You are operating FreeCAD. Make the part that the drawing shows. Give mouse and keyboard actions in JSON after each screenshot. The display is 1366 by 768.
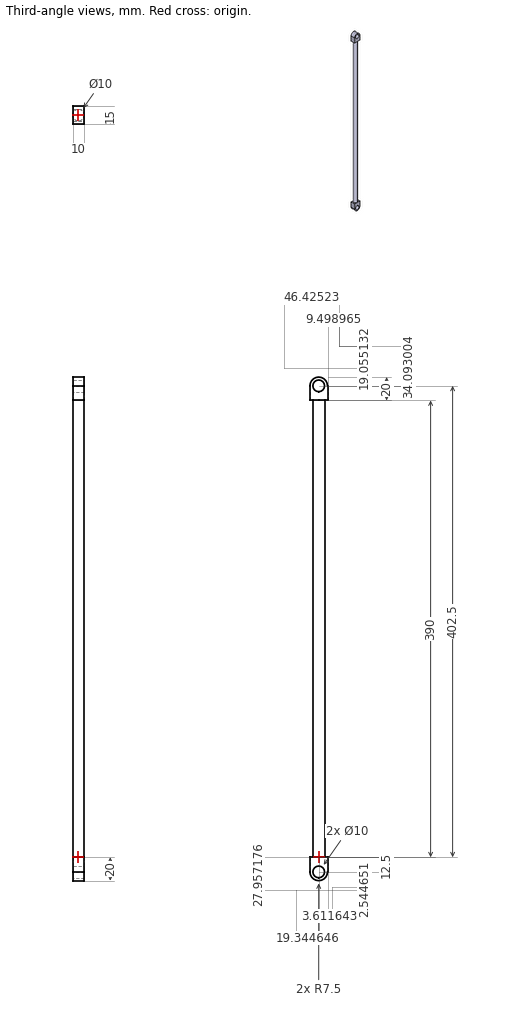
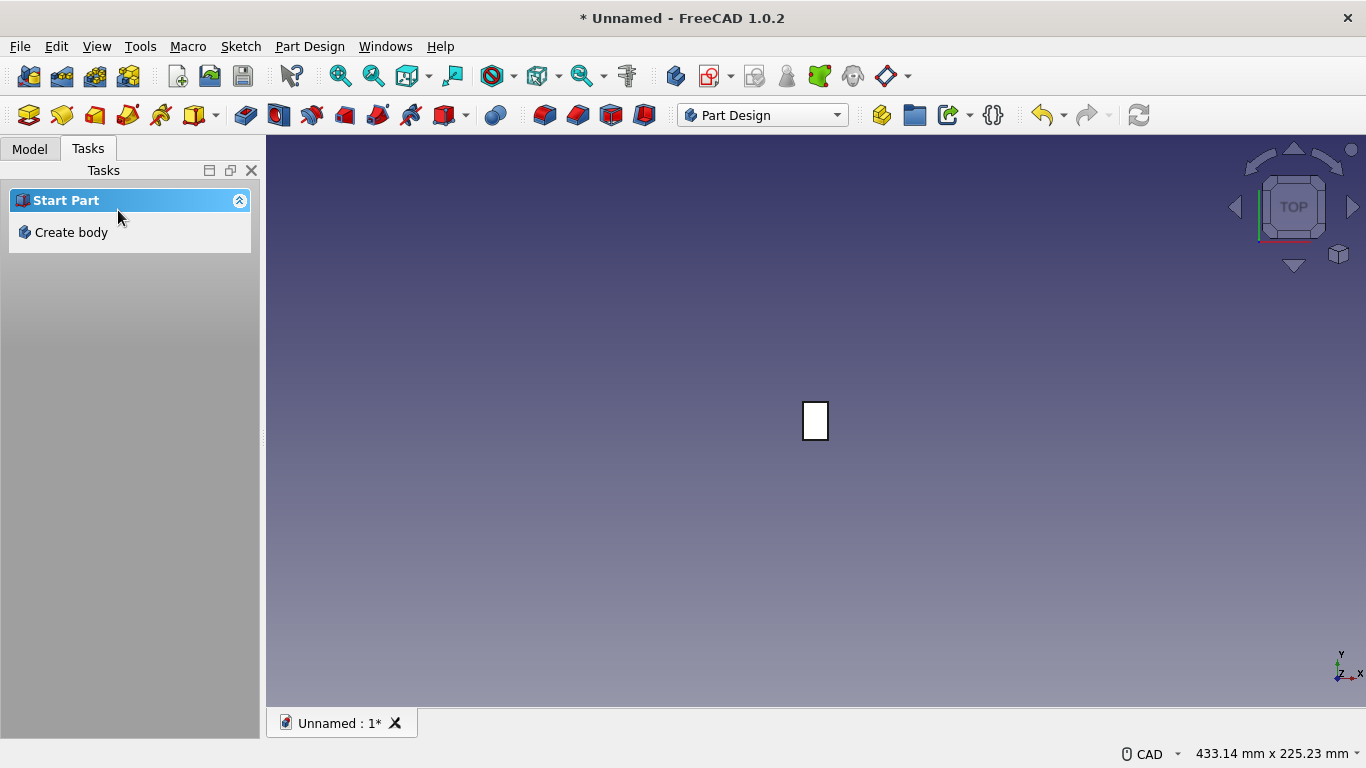
{"action": "left_click", "coordinate": [341, 76]}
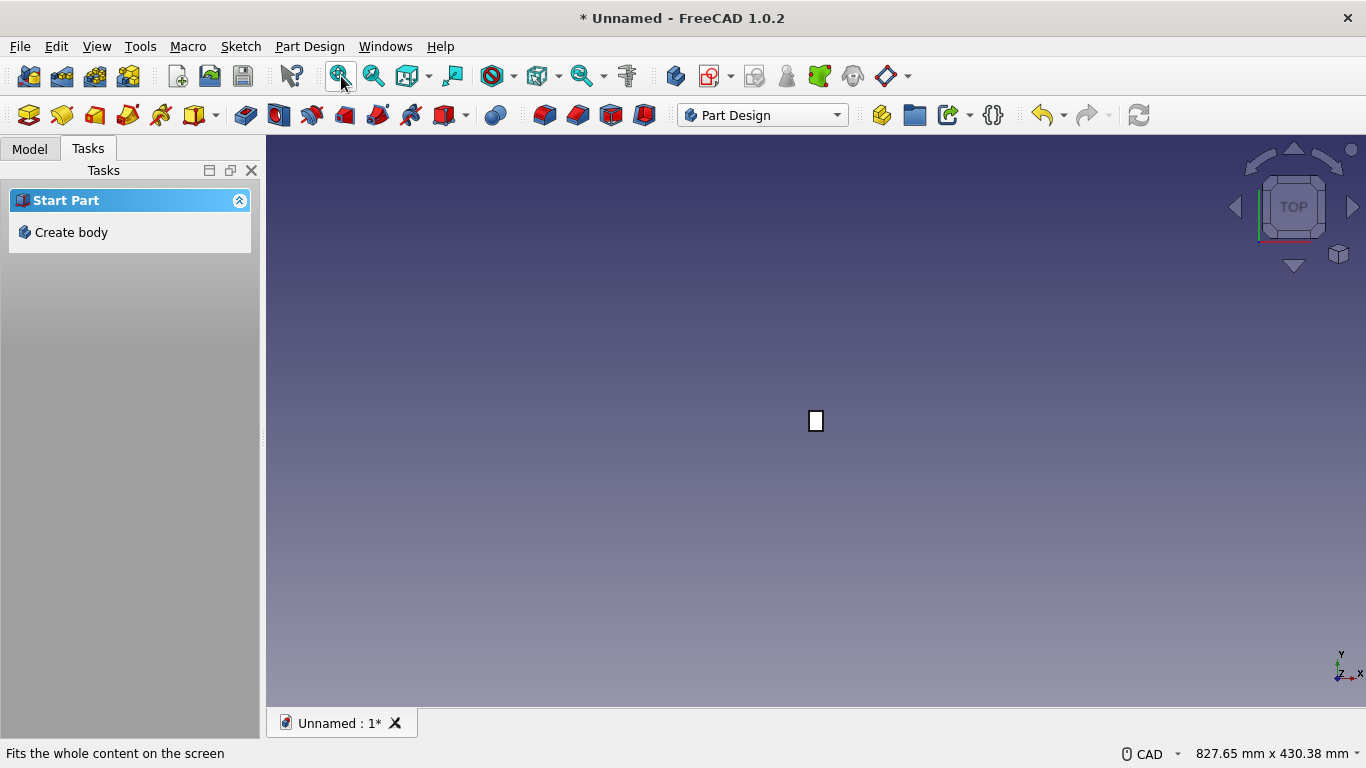
{"action": "key", "text": "0"}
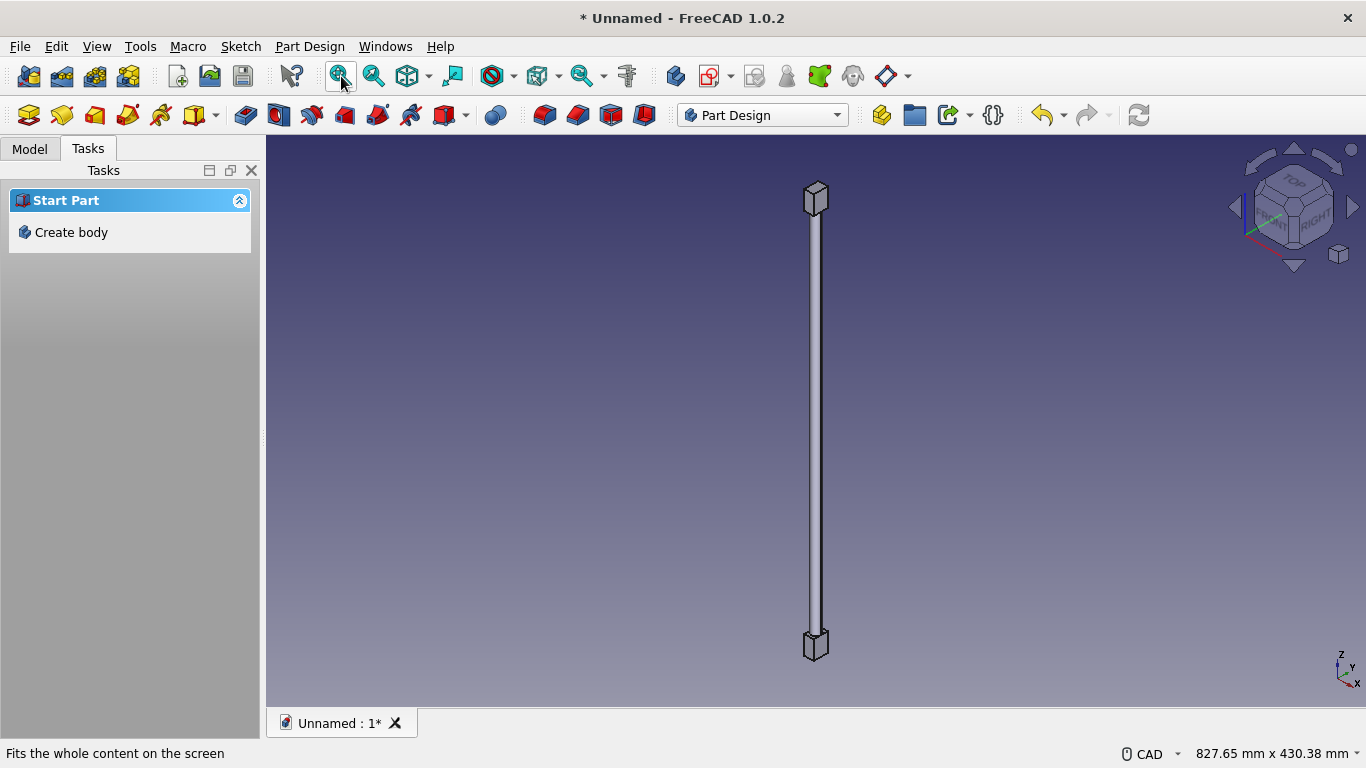
{"action": "left_click", "coordinate": [823, 199]}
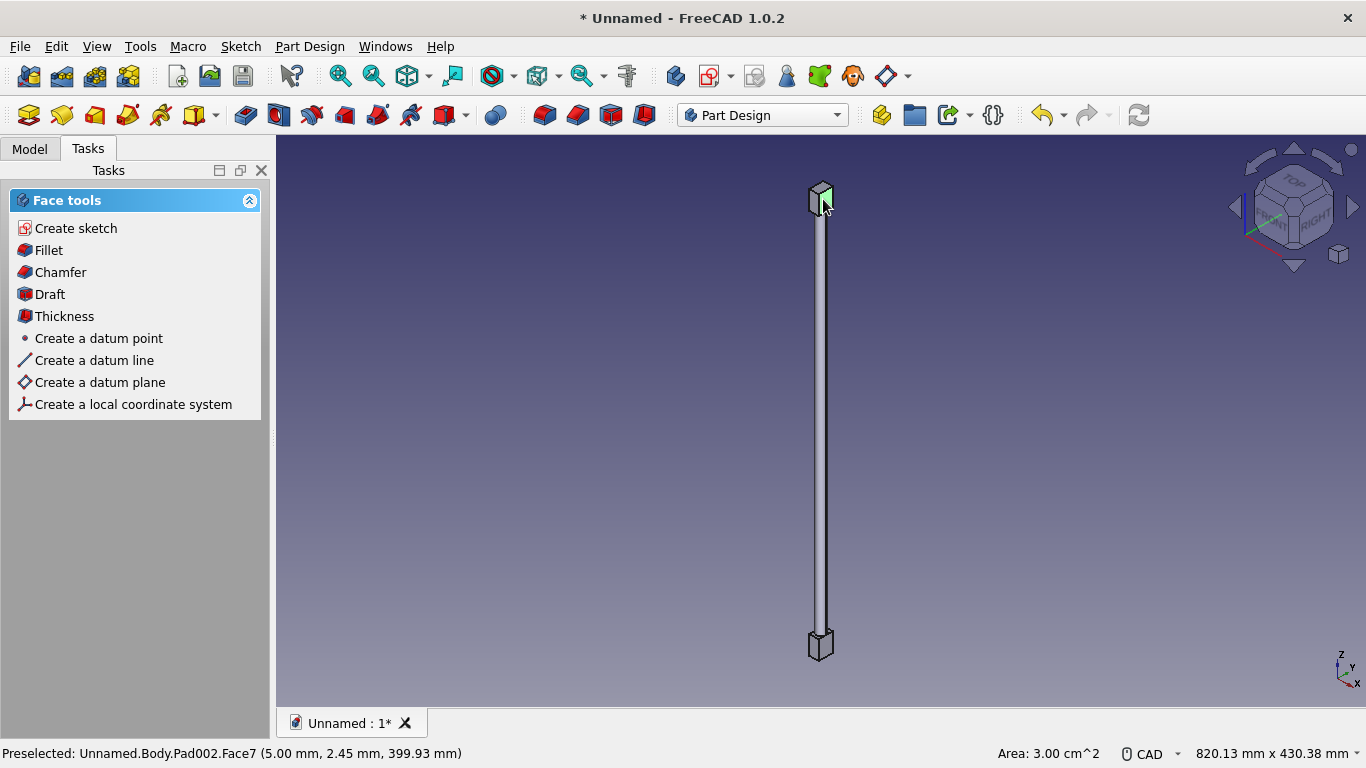
{"action": "left_click", "coordinate": [708, 76]}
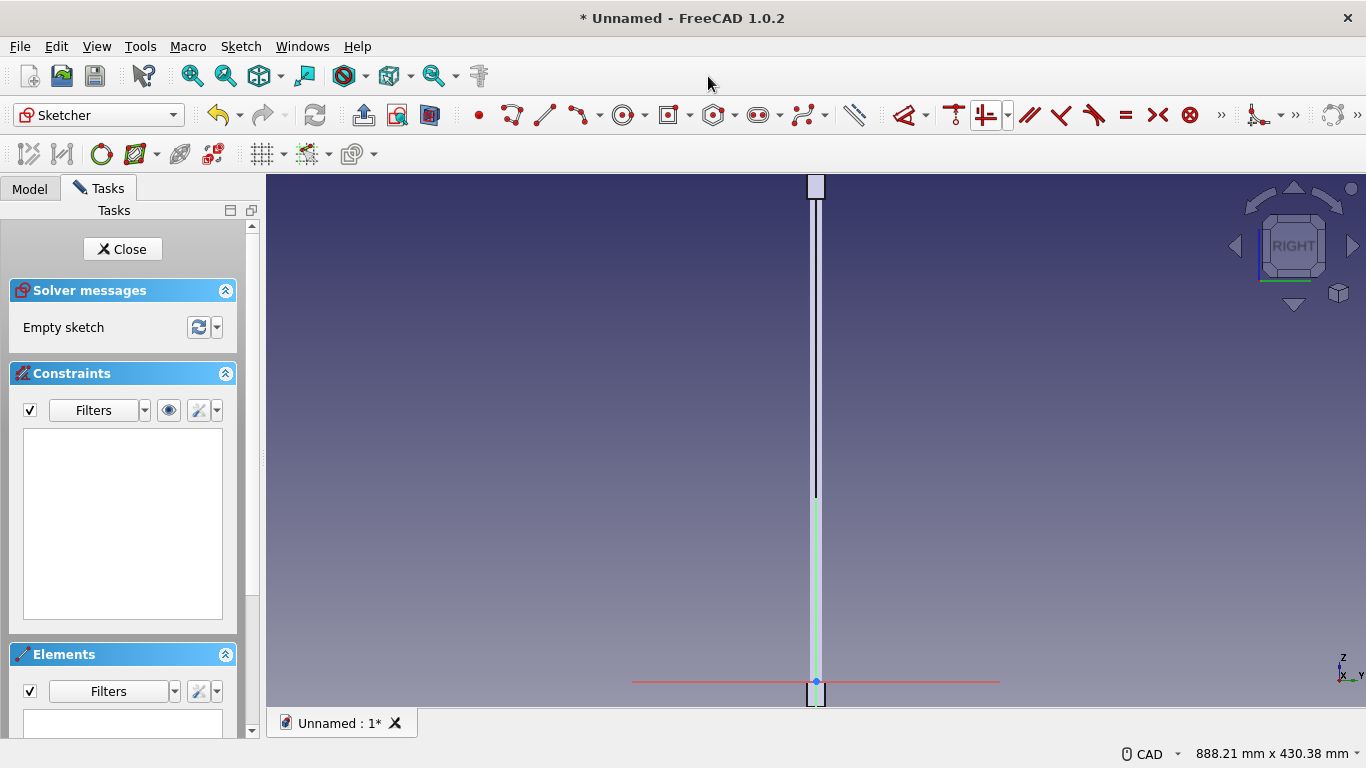
{"action": "scroll", "coordinate": [674, 455], "scroll_direction": "down", "scroll_amount": 3}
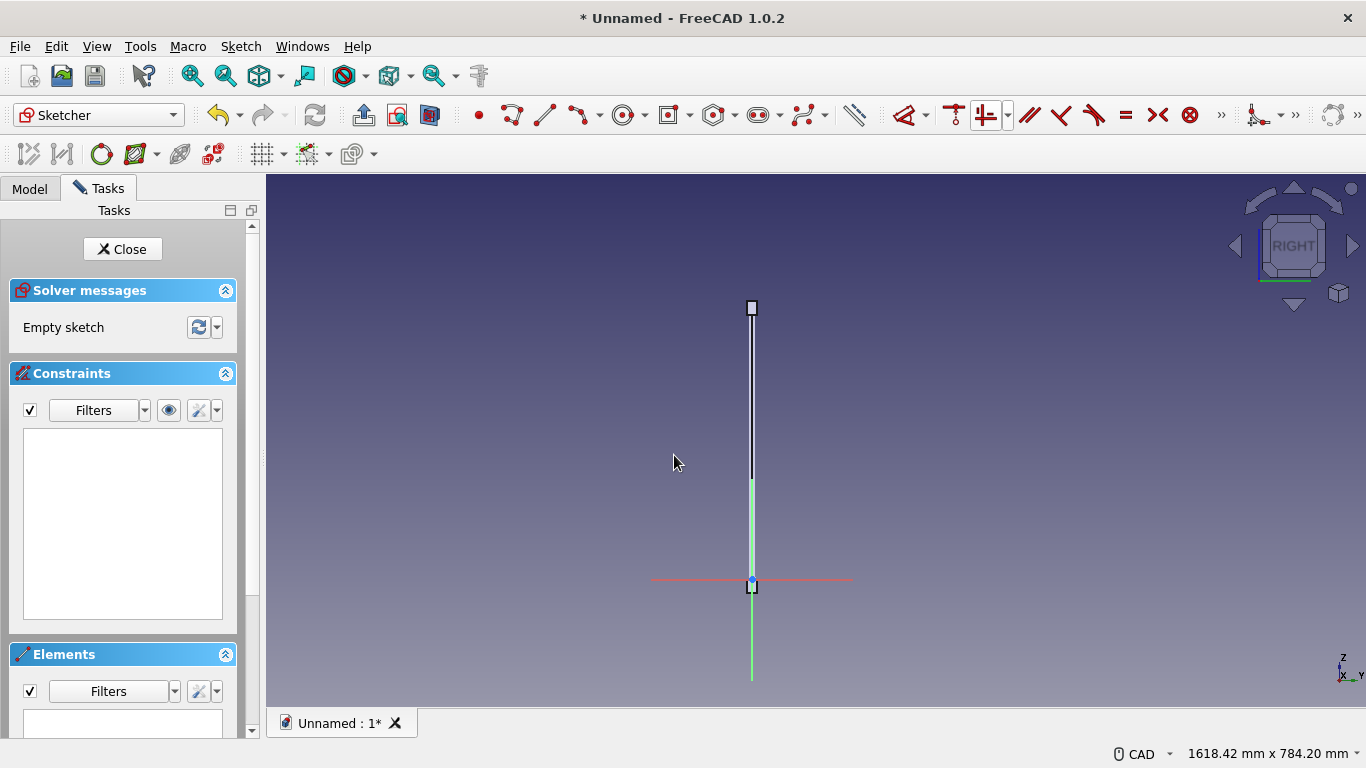
{"action": "left_click", "coordinate": [512, 116]}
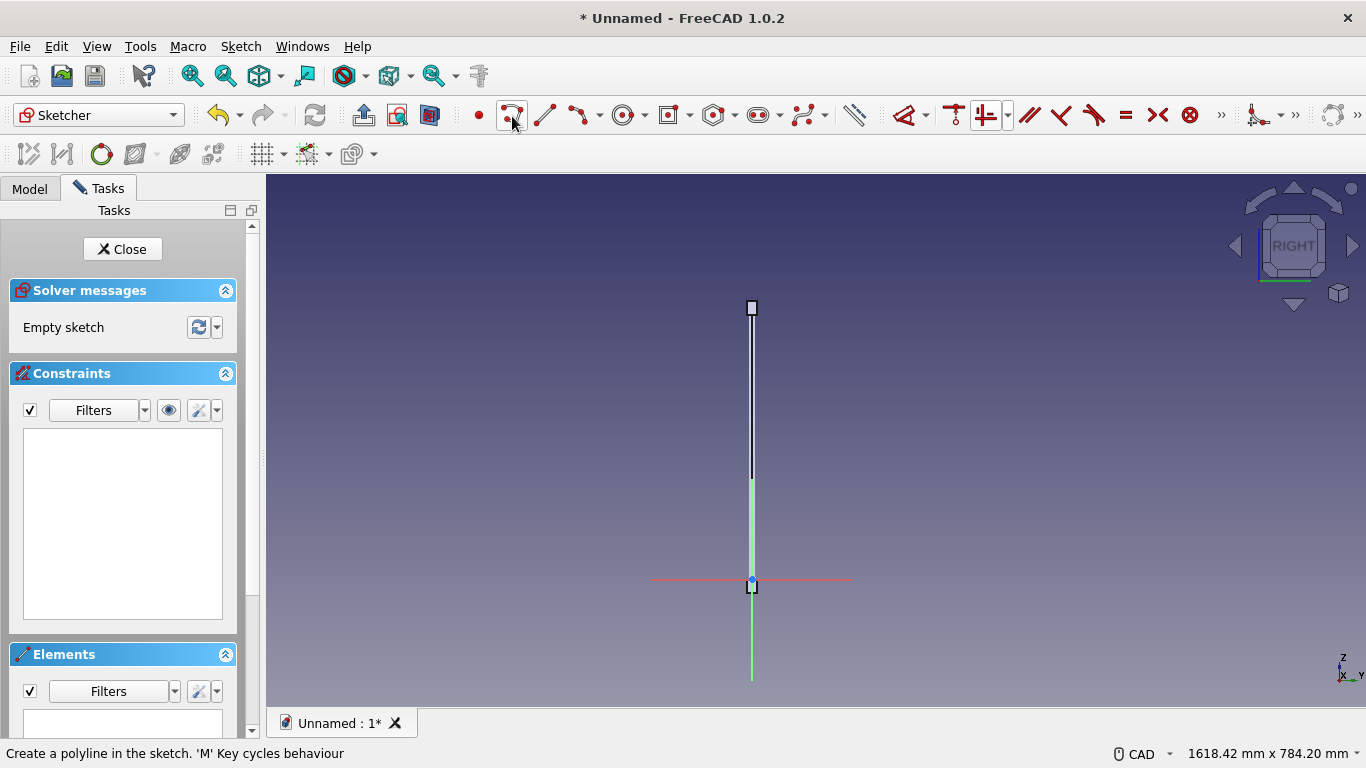
{"action": "scroll", "coordinate": [747, 588], "scroll_direction": "up", "scroll_amount": 6}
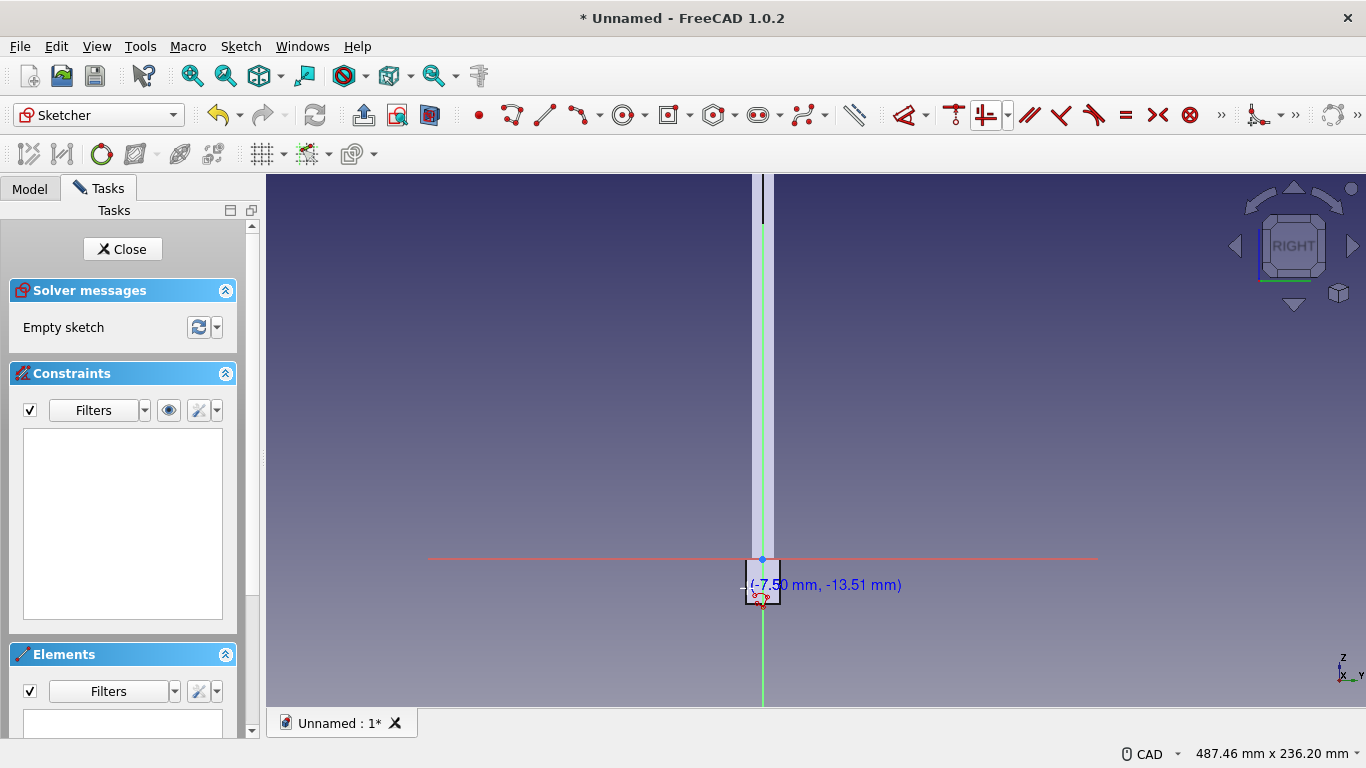
{"action": "left_click", "coordinate": [746, 587]}
{"action": "left_click", "coordinate": [719, 622]}
{"action": "left_click", "coordinate": [788, 616]}
{"action": "left_click", "coordinate": [780, 587]}
{"action": "right_click", "coordinate": [780, 587]}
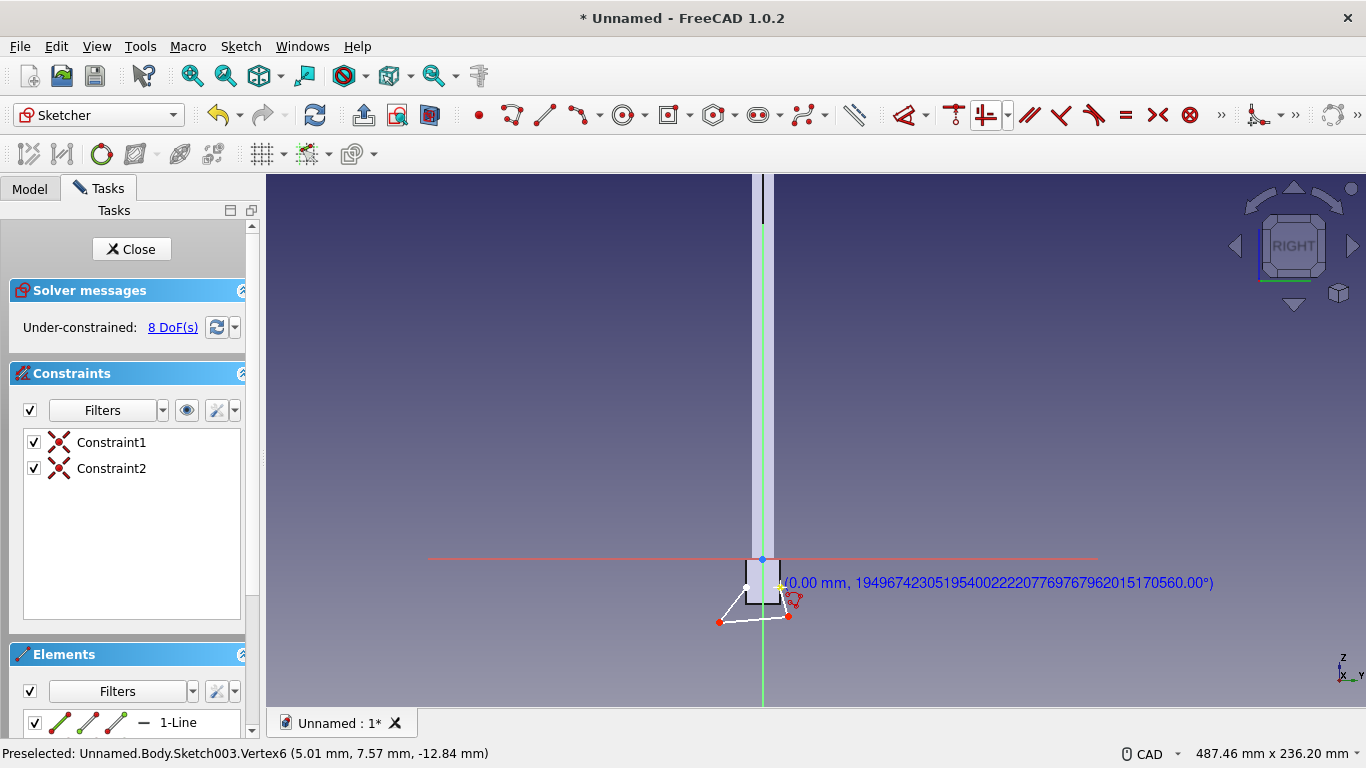
{"action": "left_click", "coordinate": [578, 116]}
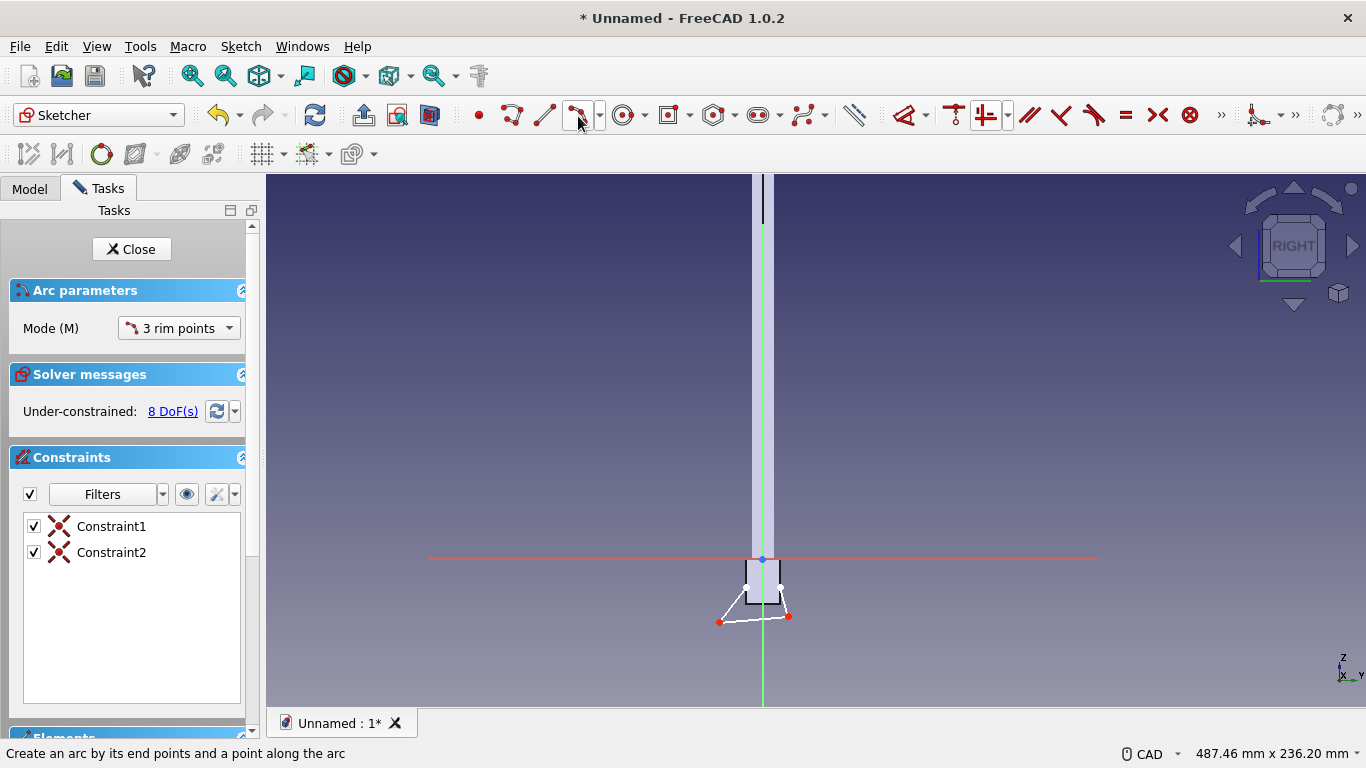
{"action": "left_click", "coordinate": [780, 588]}
{"action": "left_click", "coordinate": [746, 588]}